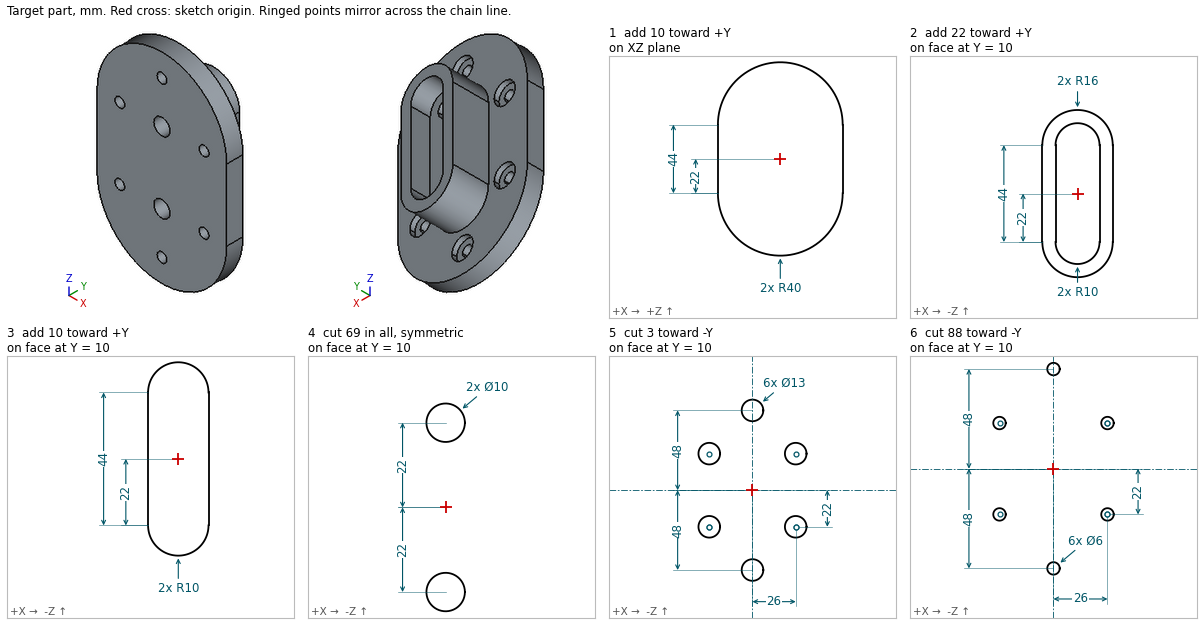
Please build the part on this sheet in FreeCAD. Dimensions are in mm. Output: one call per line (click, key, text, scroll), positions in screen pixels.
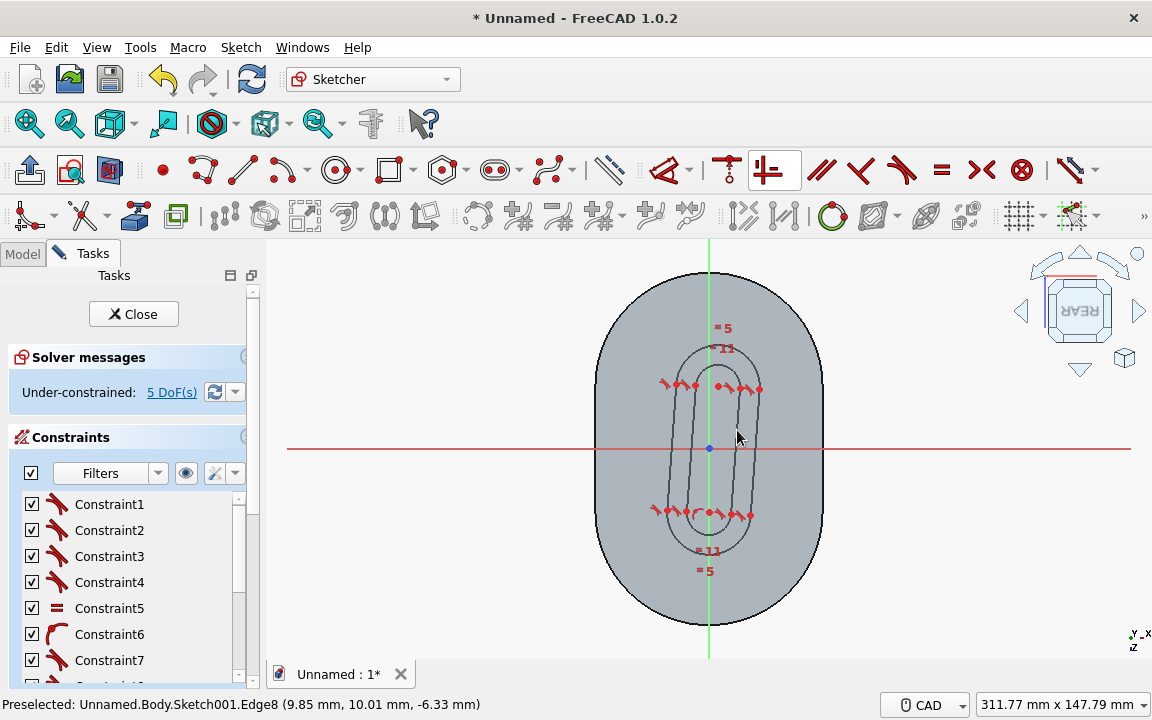
click(670, 472)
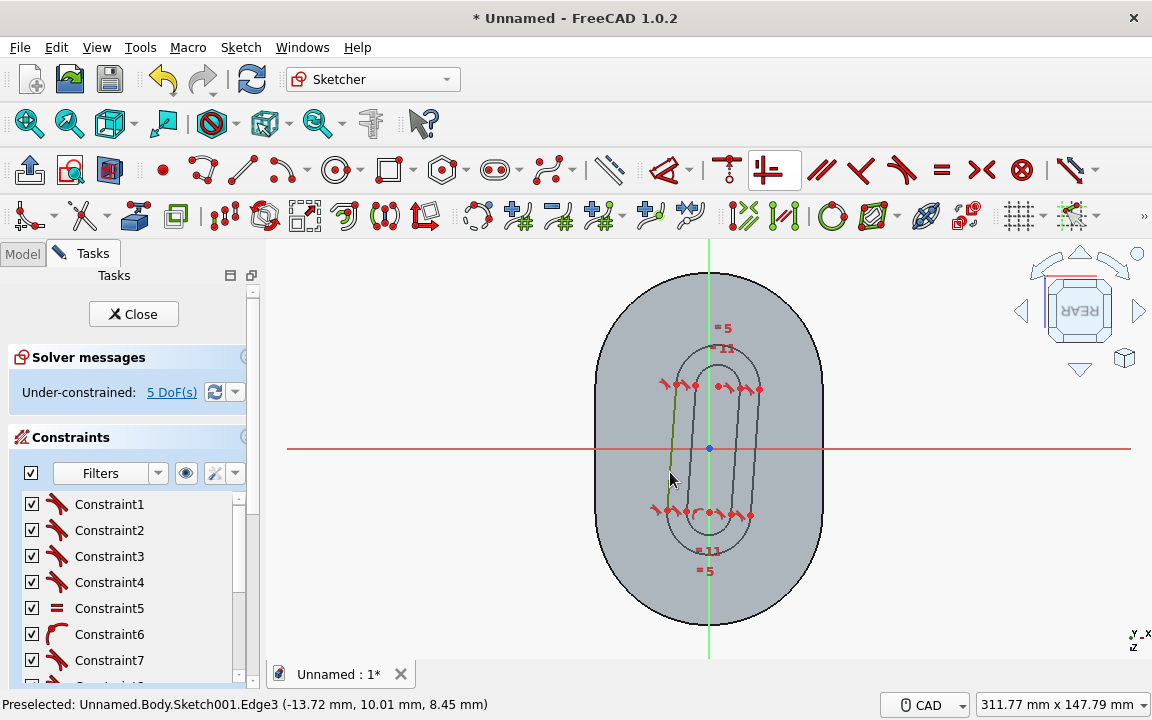
click(796, 170)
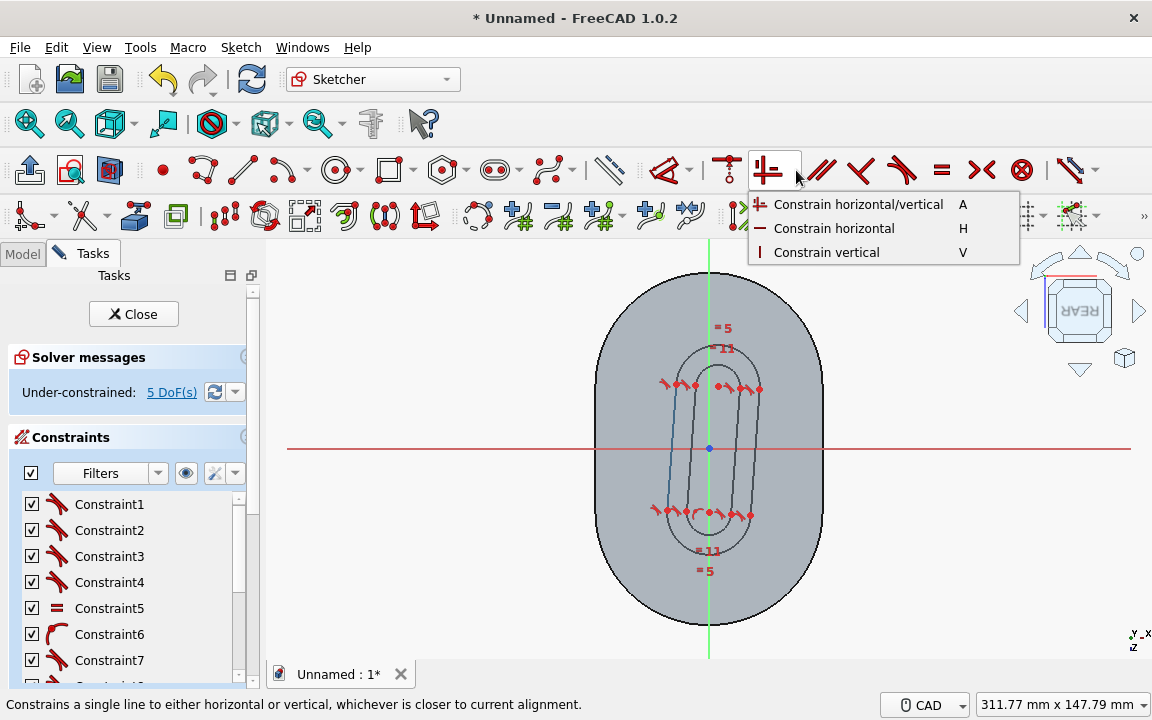
click(884, 252)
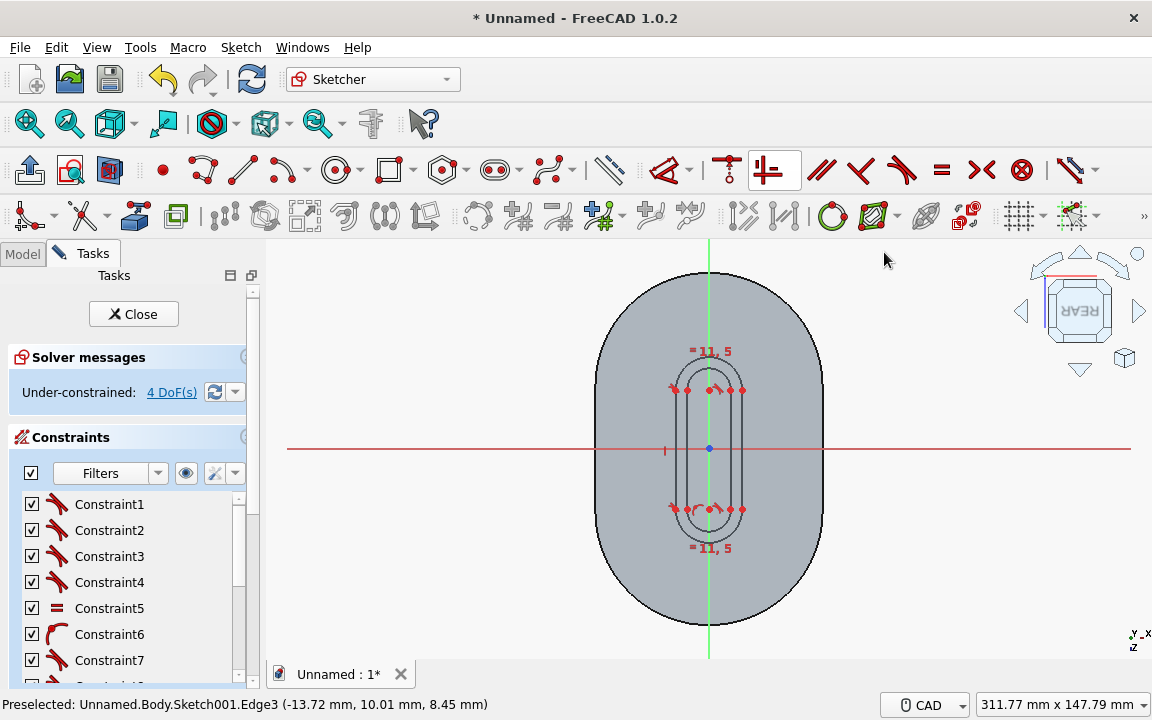
click(664, 170)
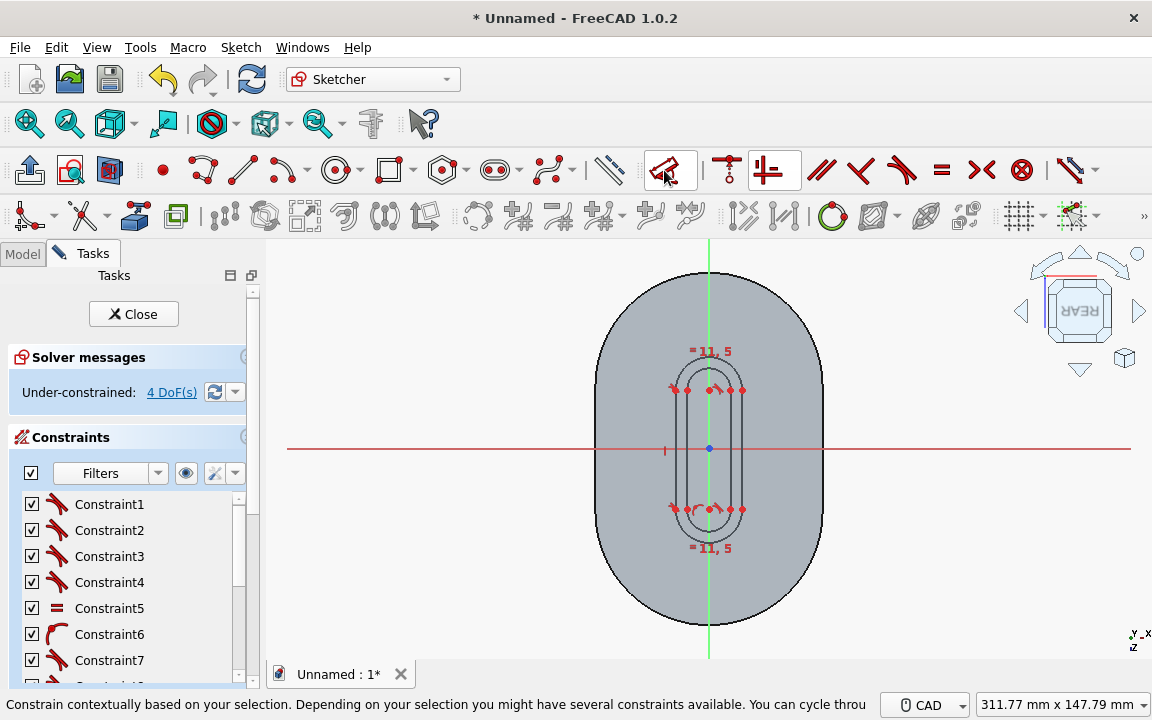
scroll(690, 537, up, 2)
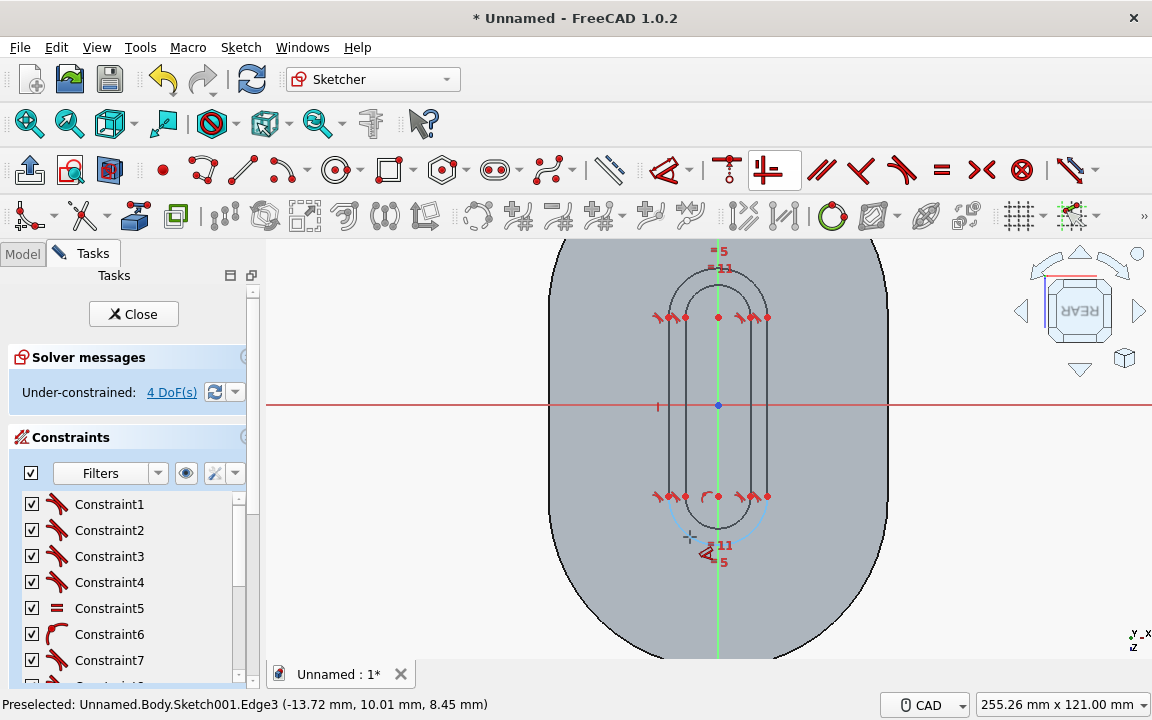
click(689, 536)
click(670, 562)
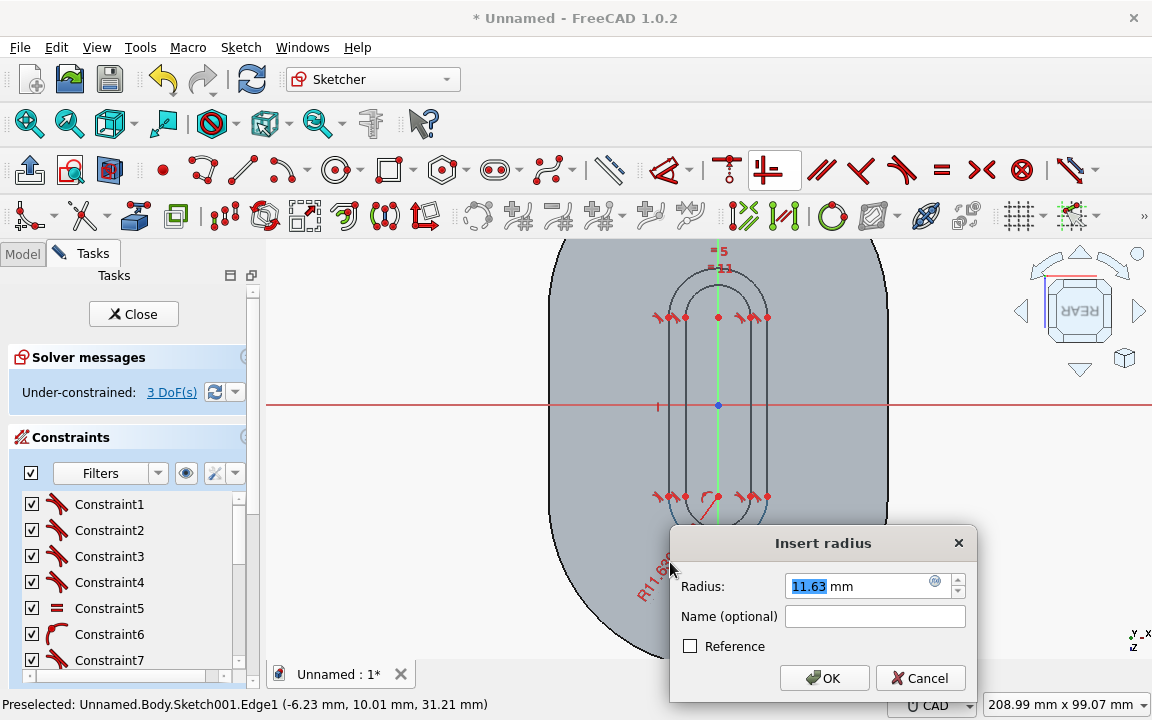
text(16)
key(Return)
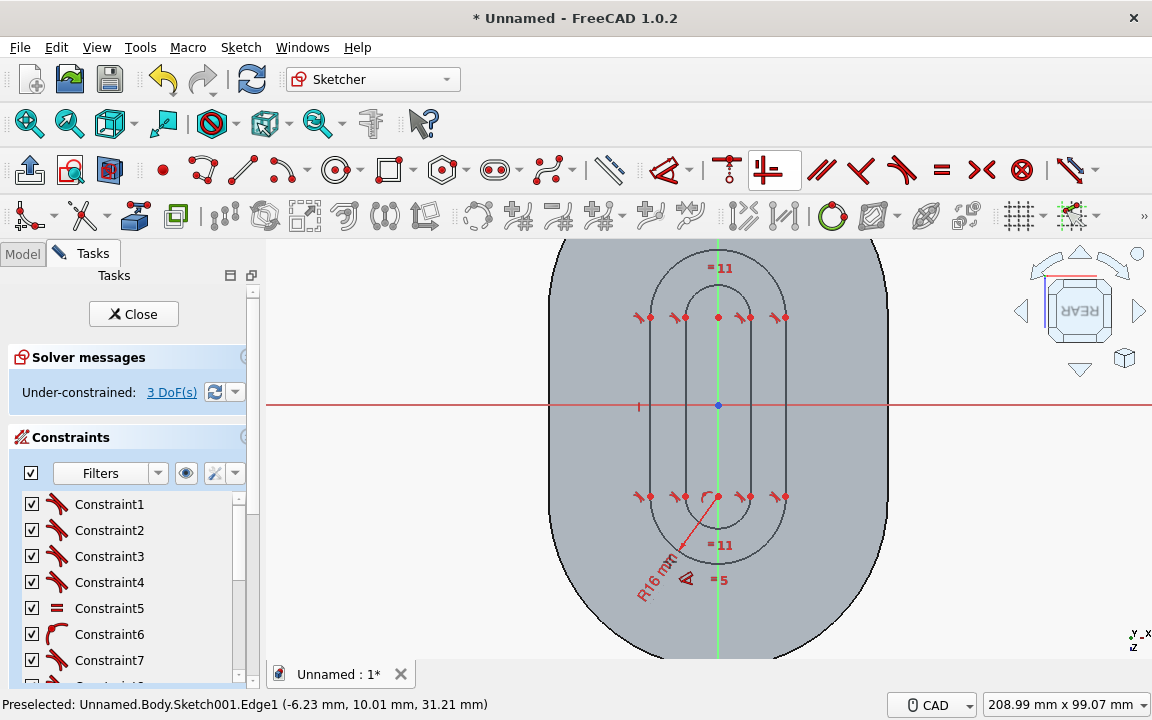
click(699, 522)
click(666, 458)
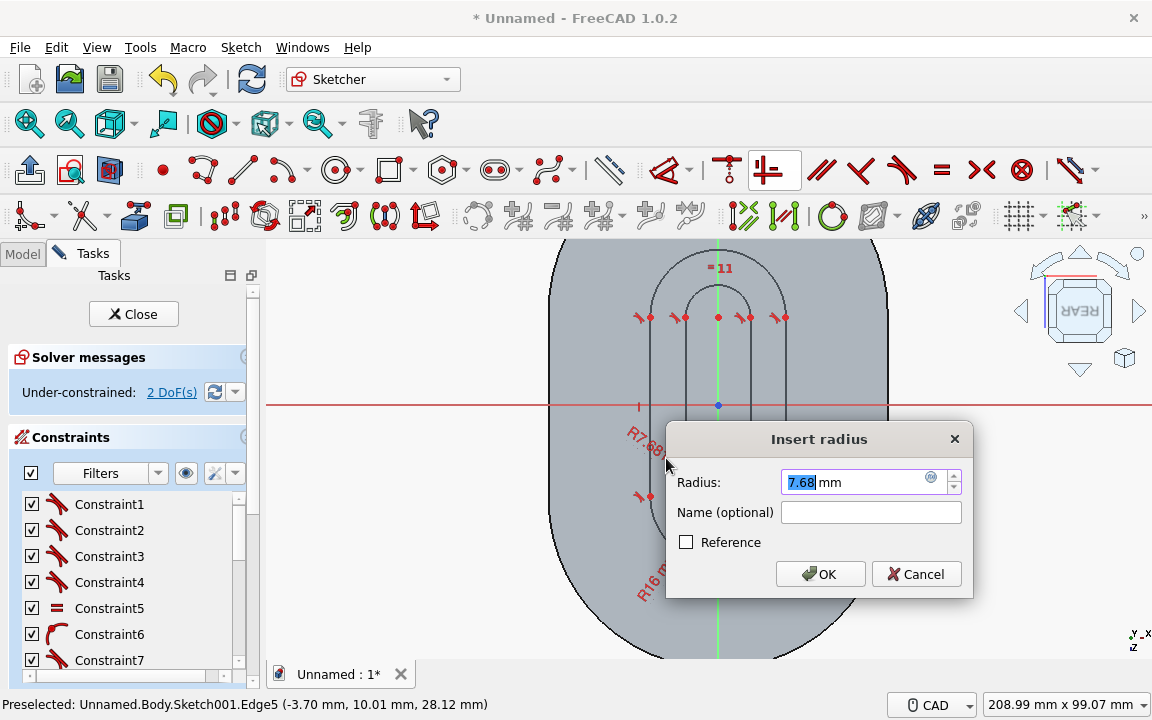
text(10)
key(Return)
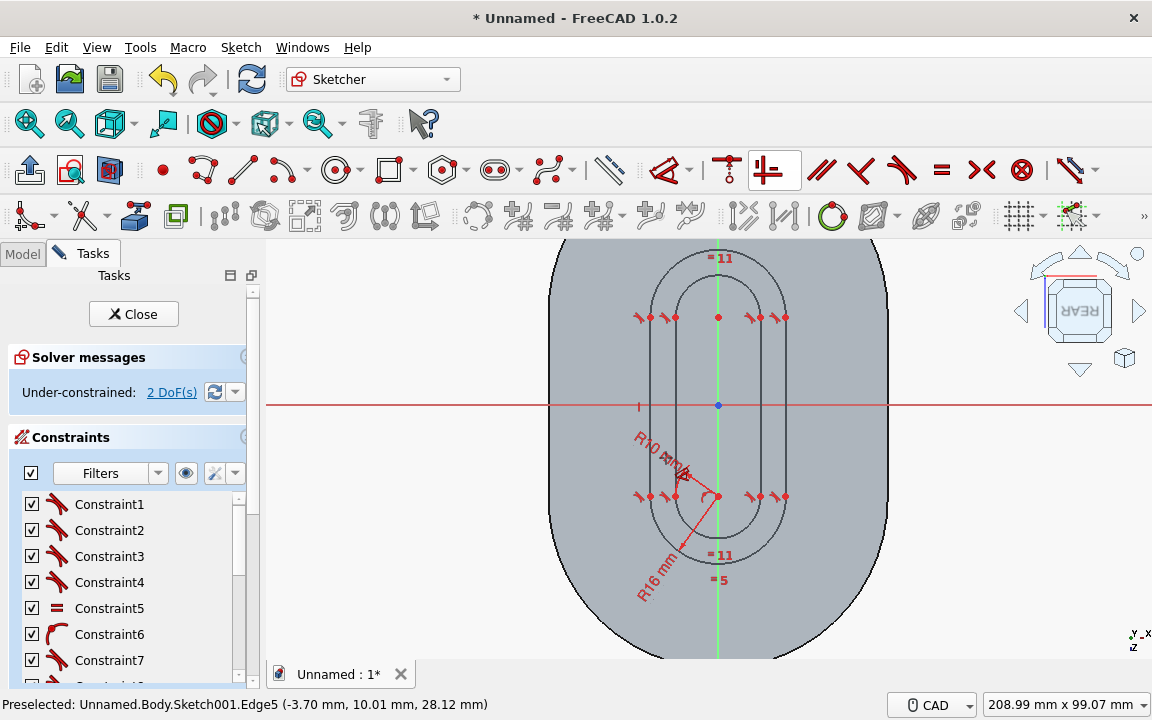
click(650, 443)
click(616, 366)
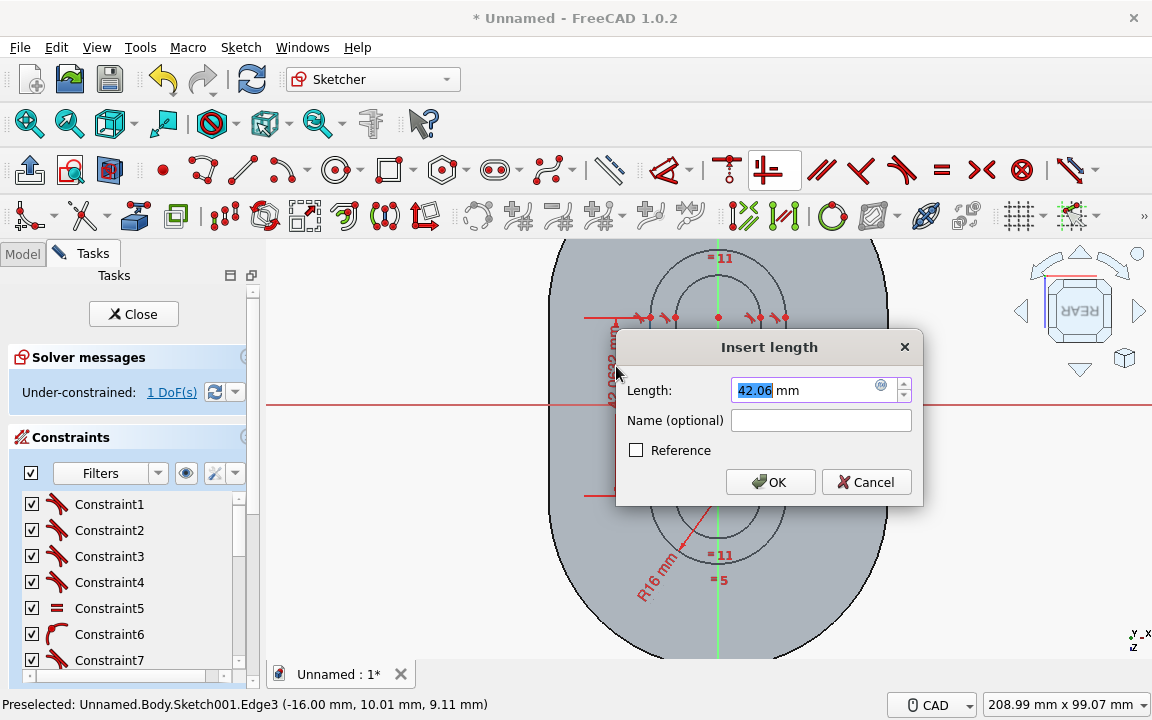
text(44)
key(Return)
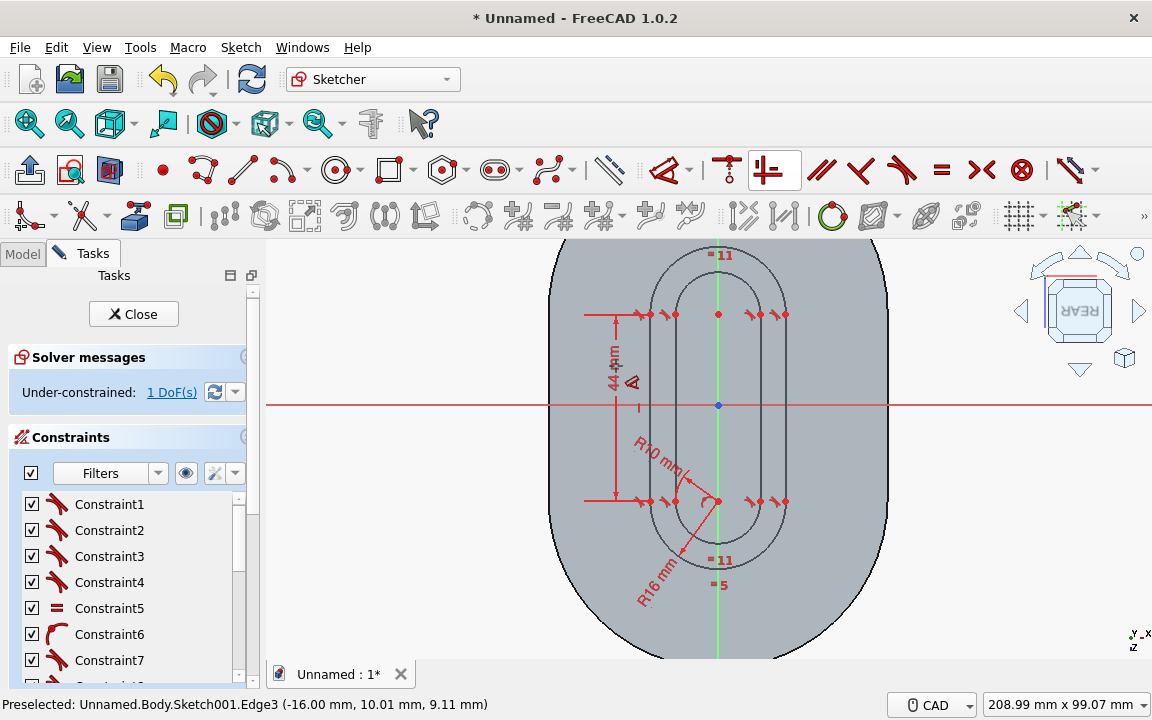
click(650, 501)
click(616, 431)